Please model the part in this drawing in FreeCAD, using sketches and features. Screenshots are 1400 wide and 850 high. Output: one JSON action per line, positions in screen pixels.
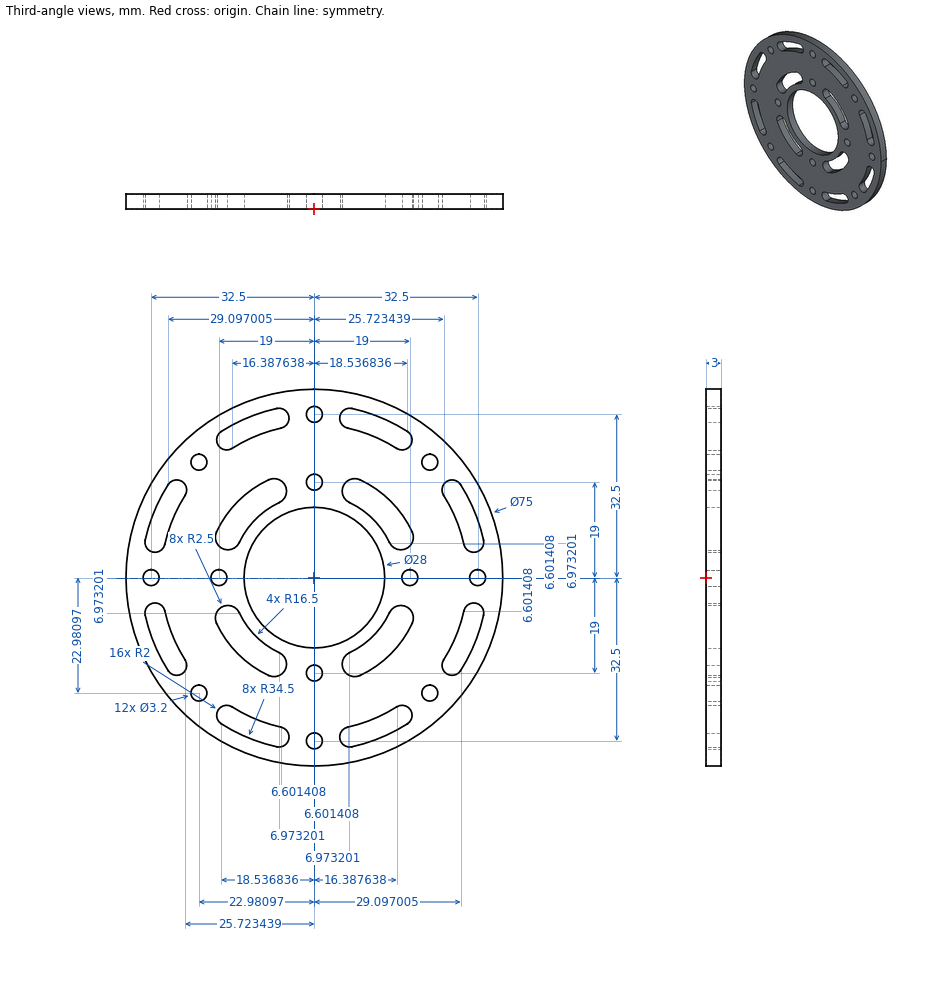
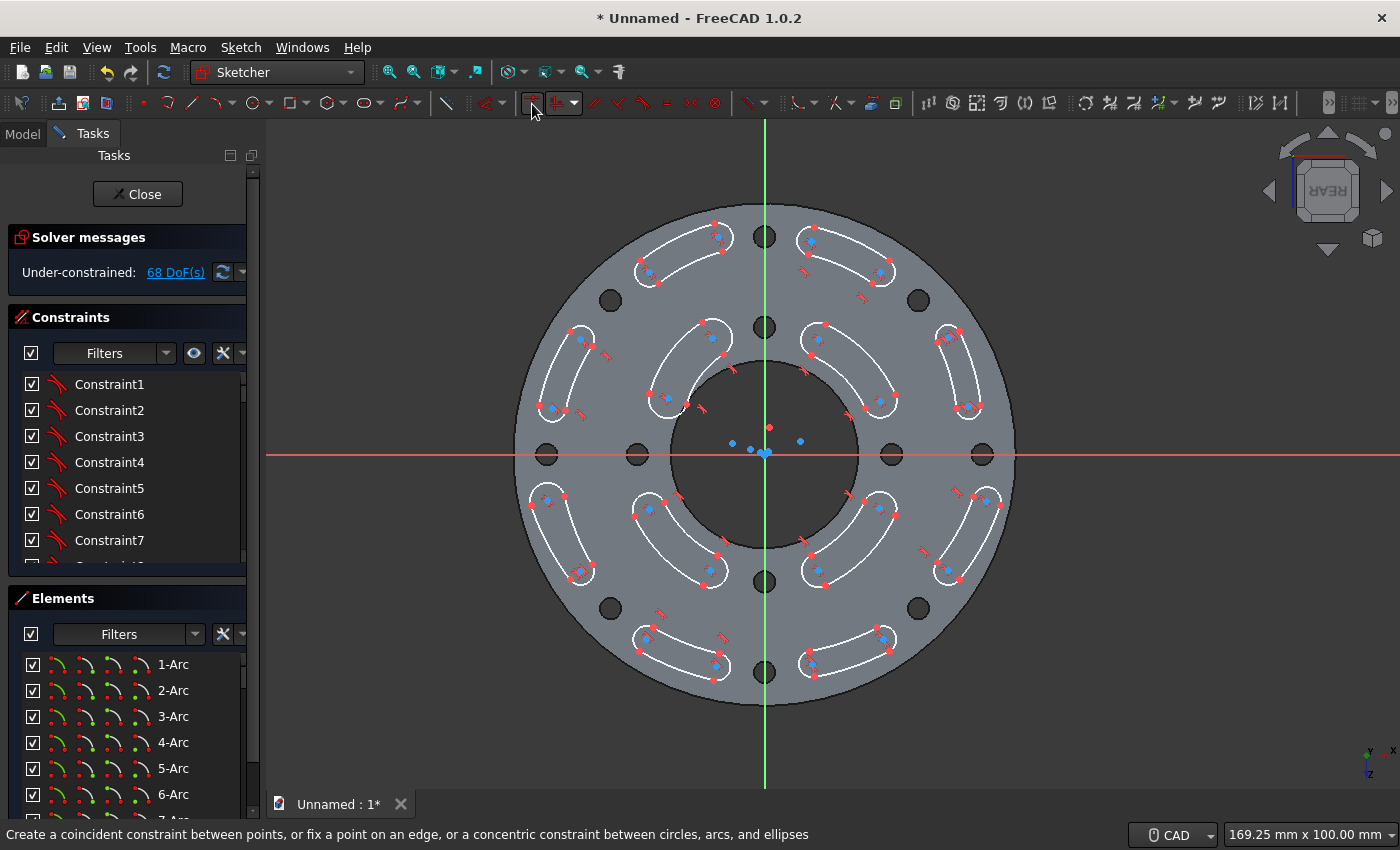
{"action": "left_click", "coordinate": [691, 232]}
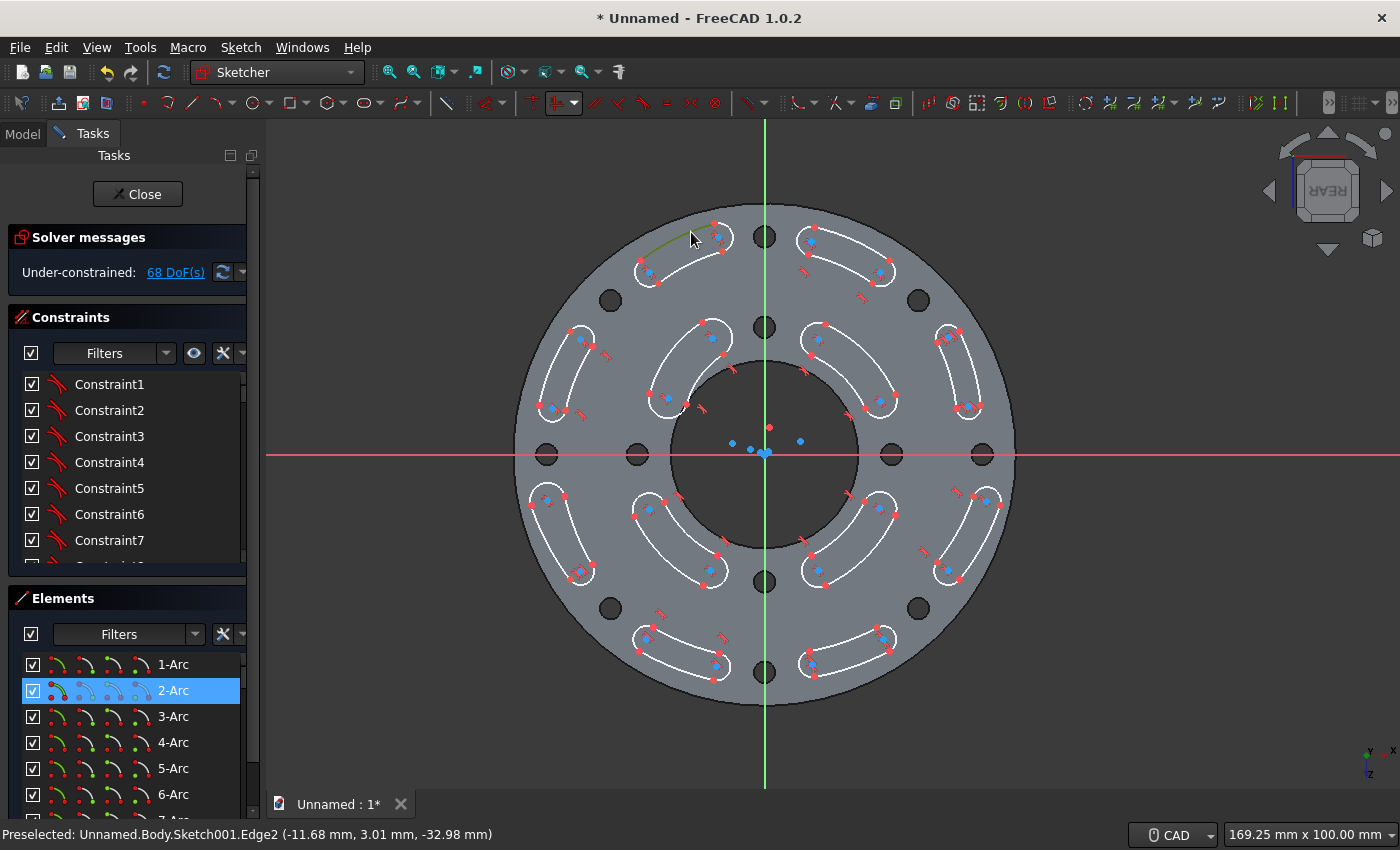
{"action": "left_click", "coordinate": [571, 518]}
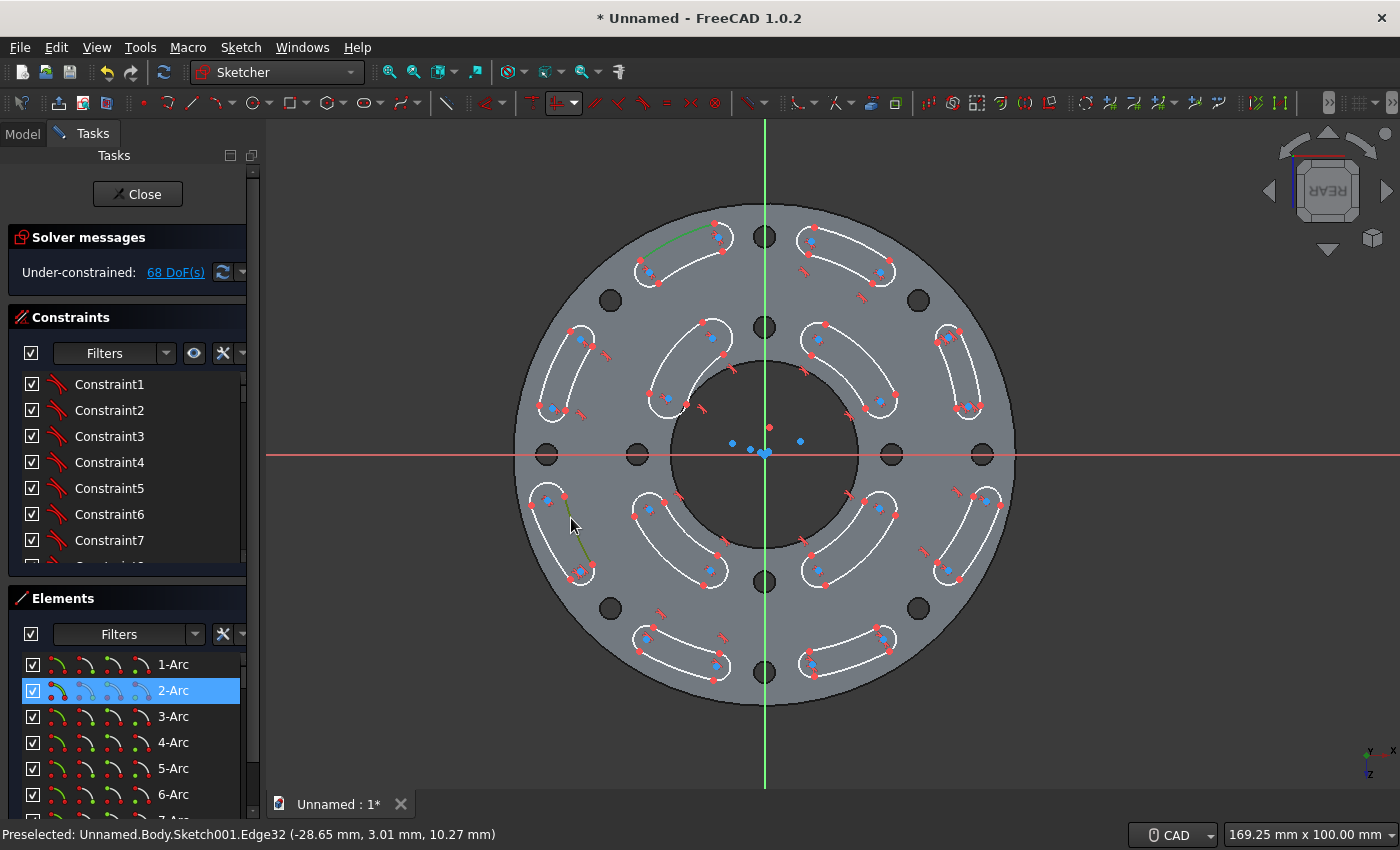
{"action": "left_click", "coordinate": [532, 104]}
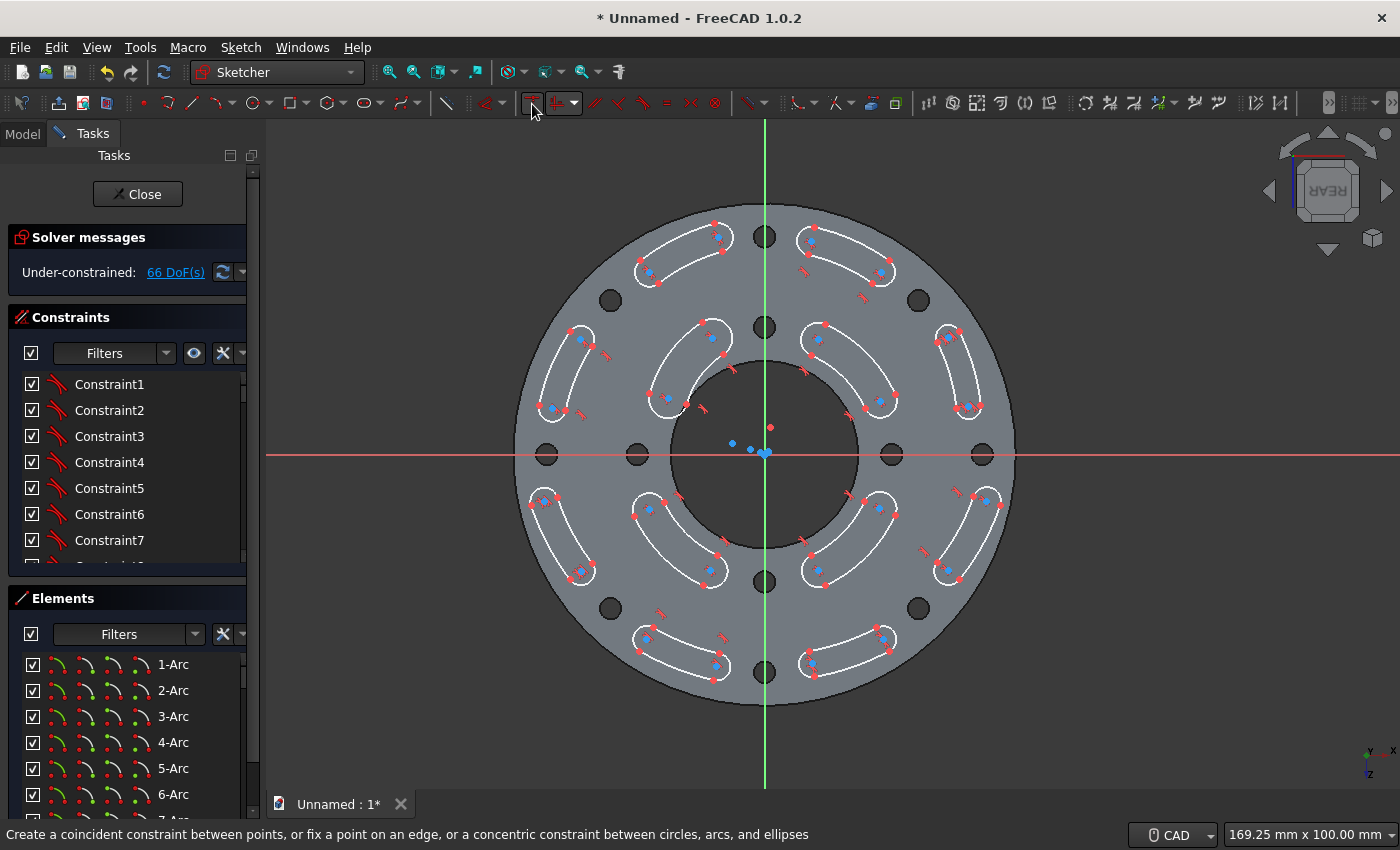
{"action": "left_click", "coordinate": [691, 232]}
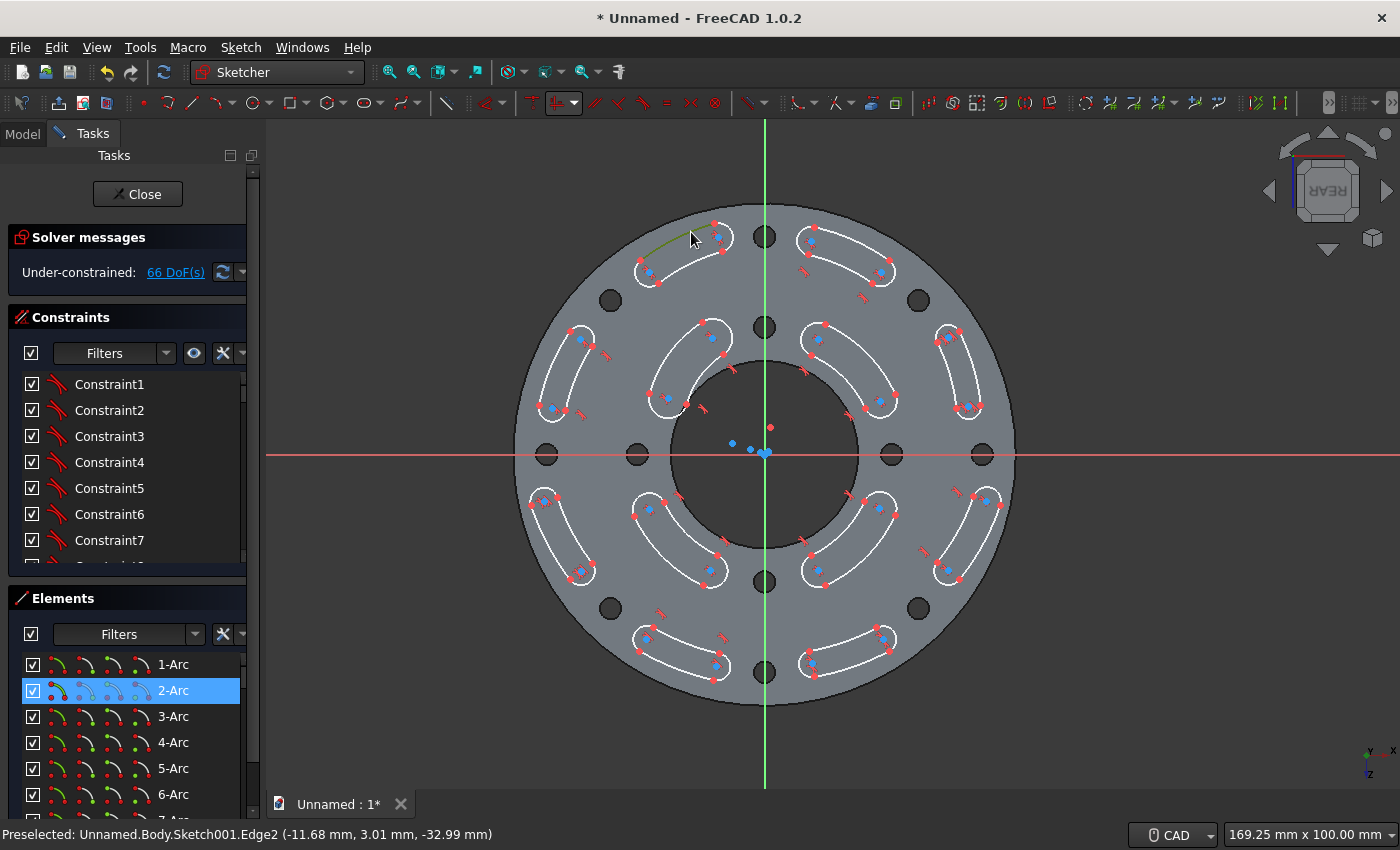
{"action": "left_click", "coordinate": [582, 365]}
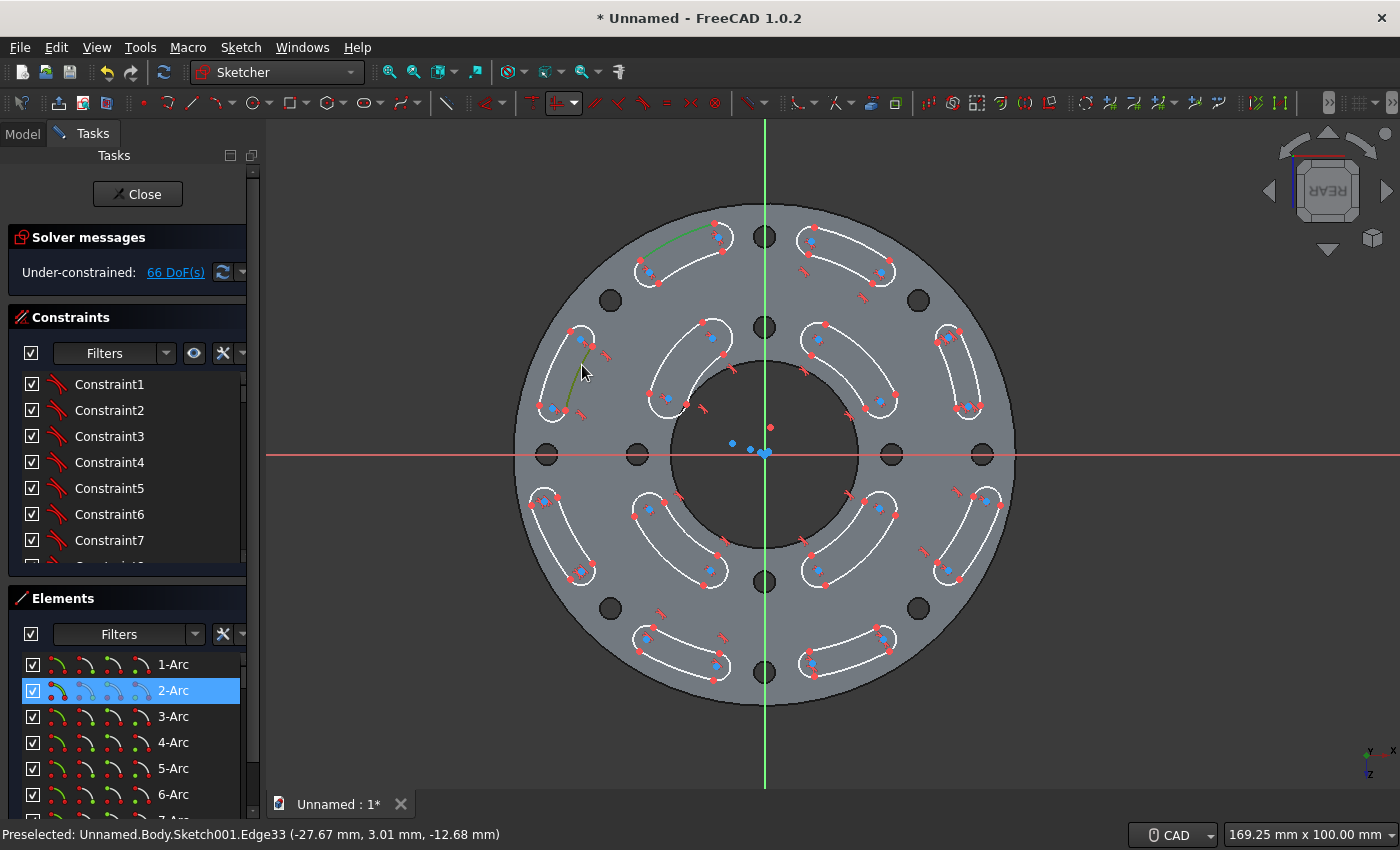
{"action": "left_click", "coordinate": [532, 104]}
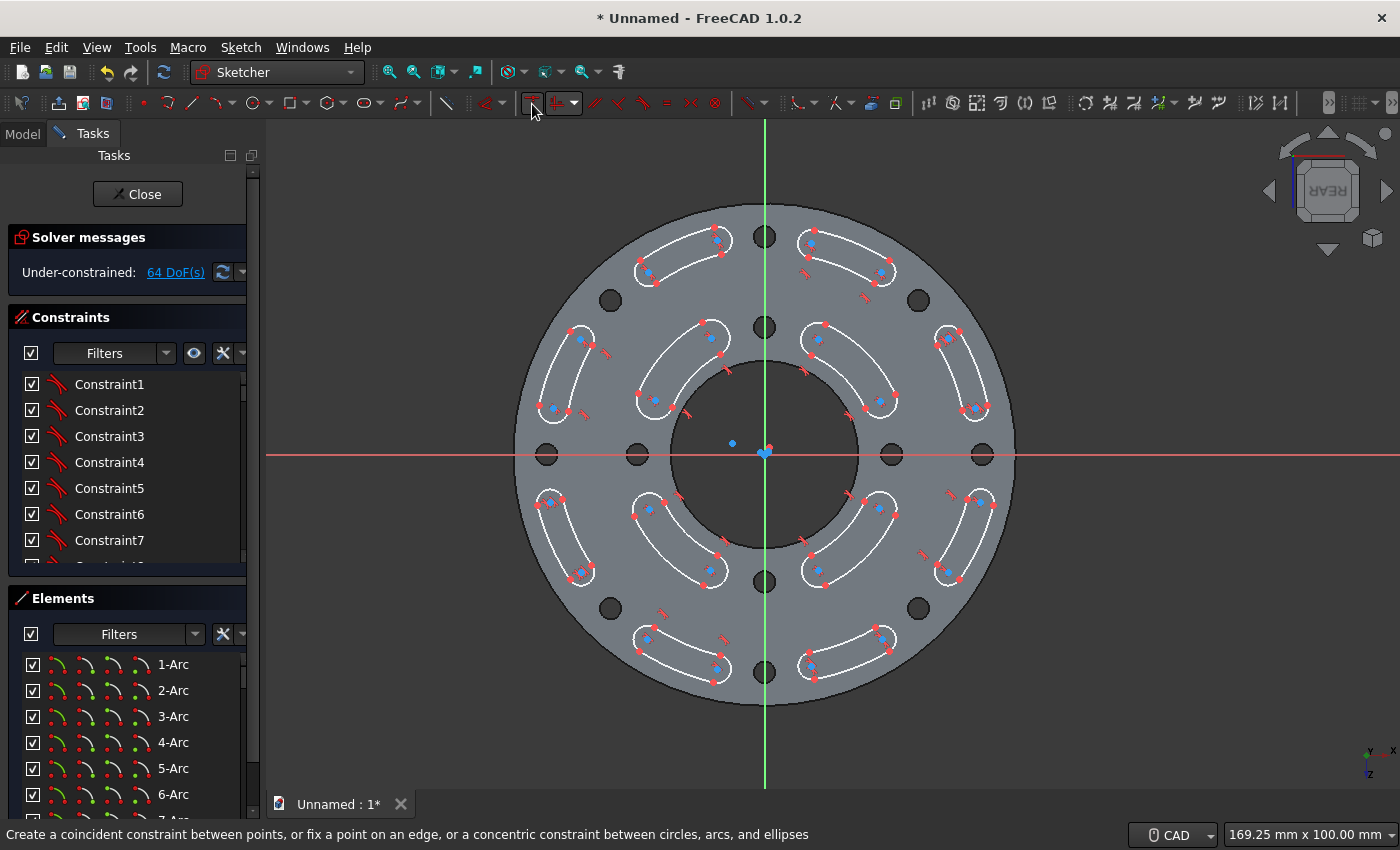
{"action": "left_click", "coordinate": [691, 234]}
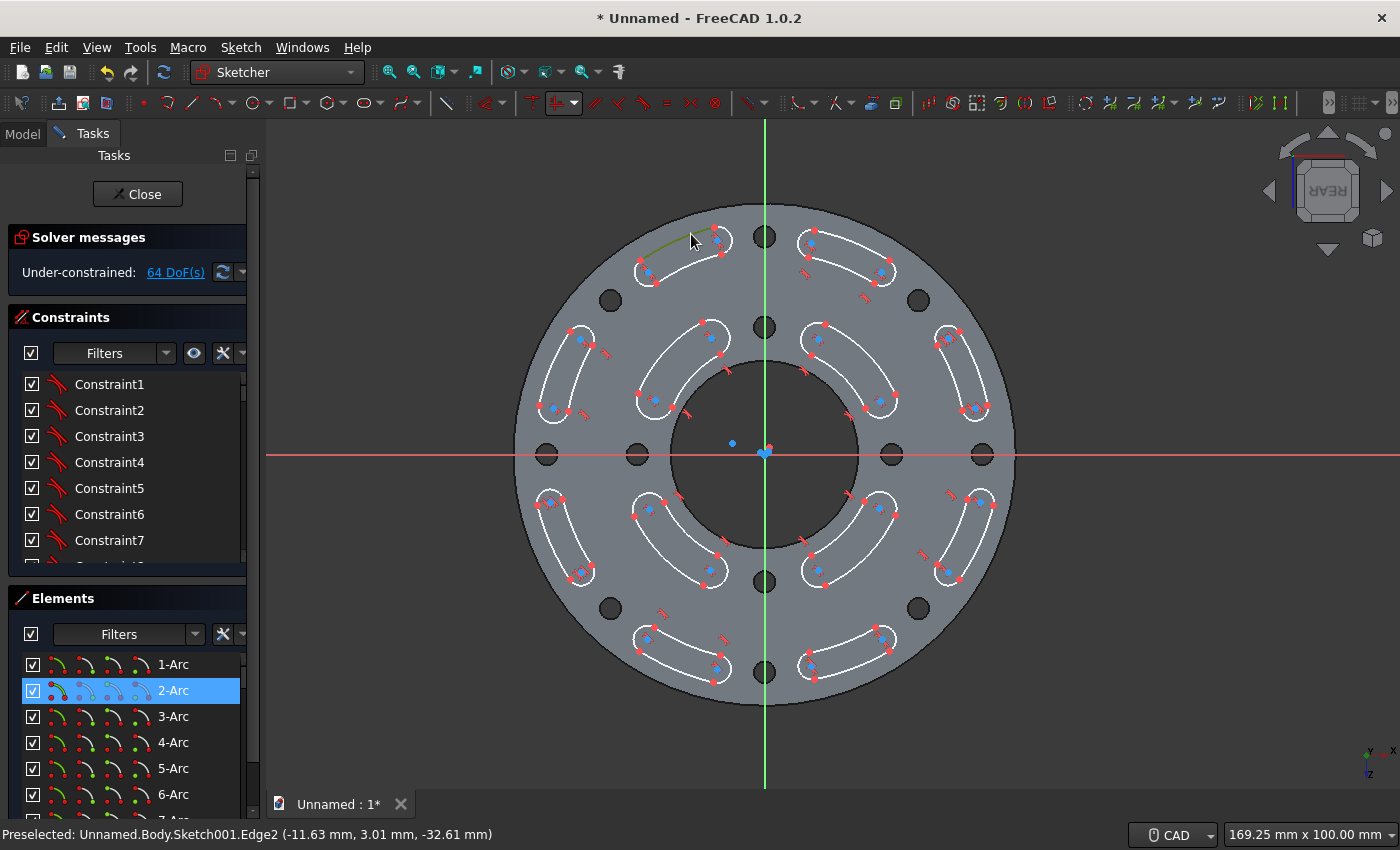
{"action": "left_click", "coordinate": [558, 352]}